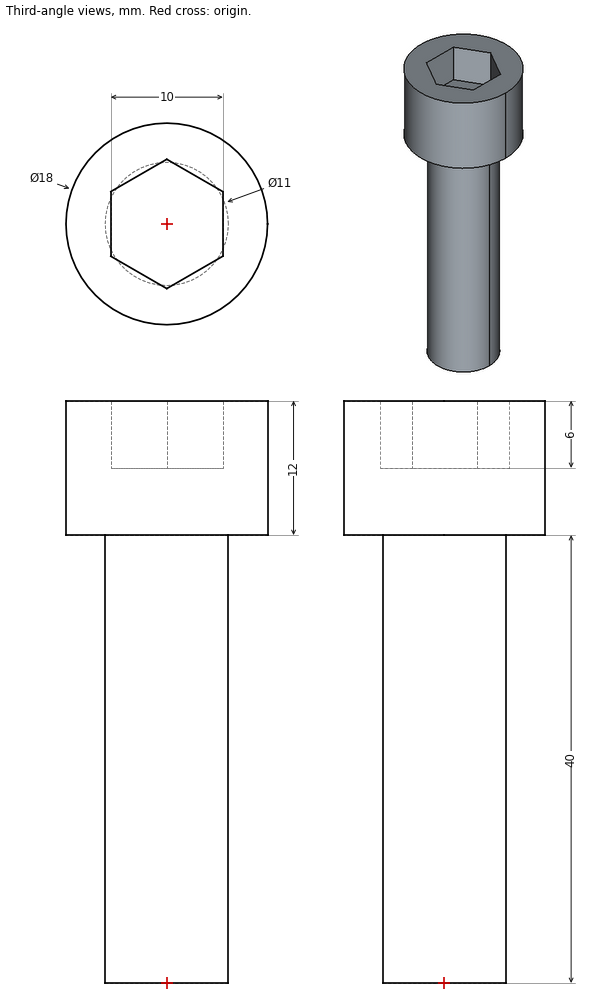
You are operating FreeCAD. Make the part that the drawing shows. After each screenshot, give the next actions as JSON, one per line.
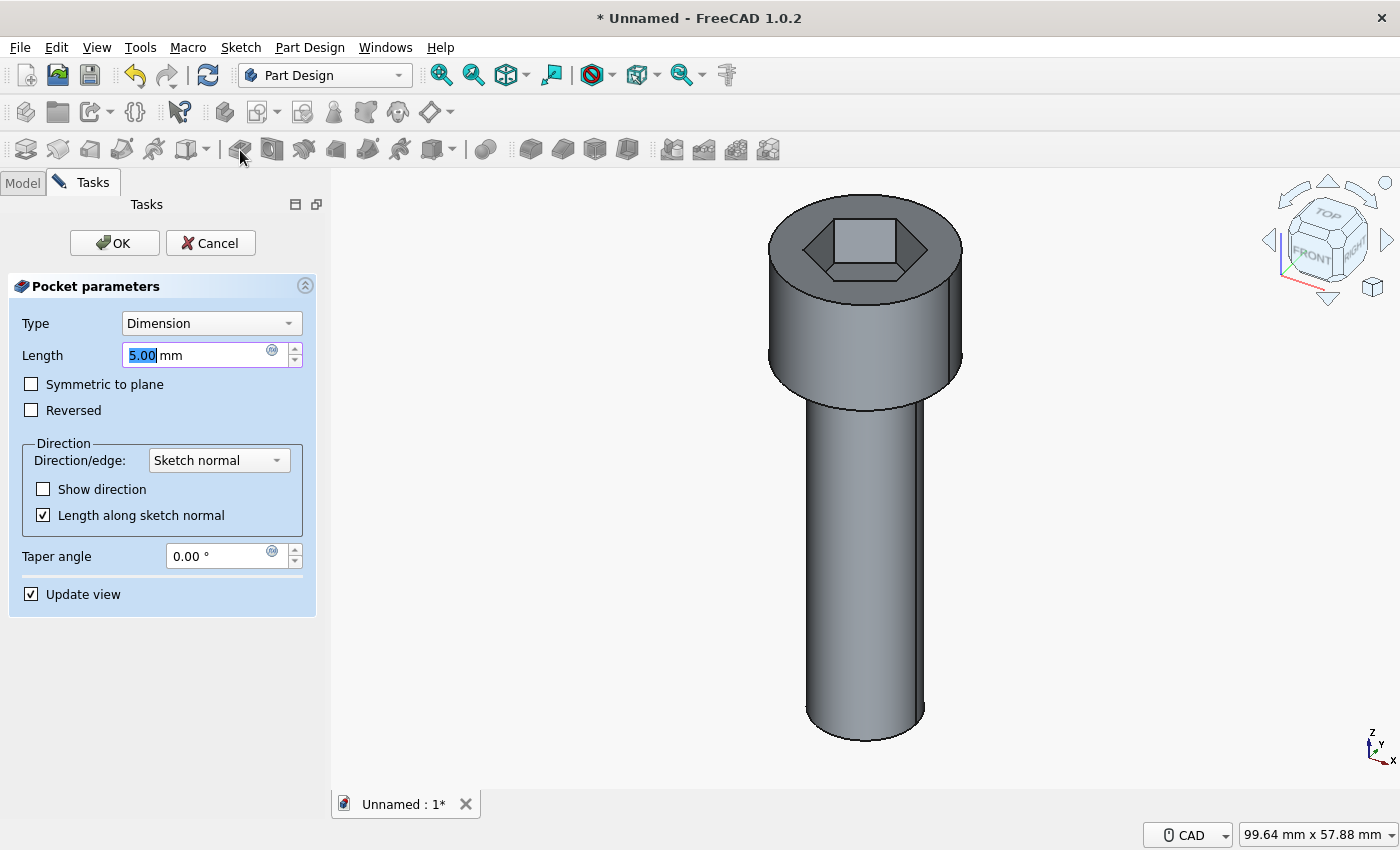
{"action": "type", "text": "6"}
{"action": "key", "text": "Tab"}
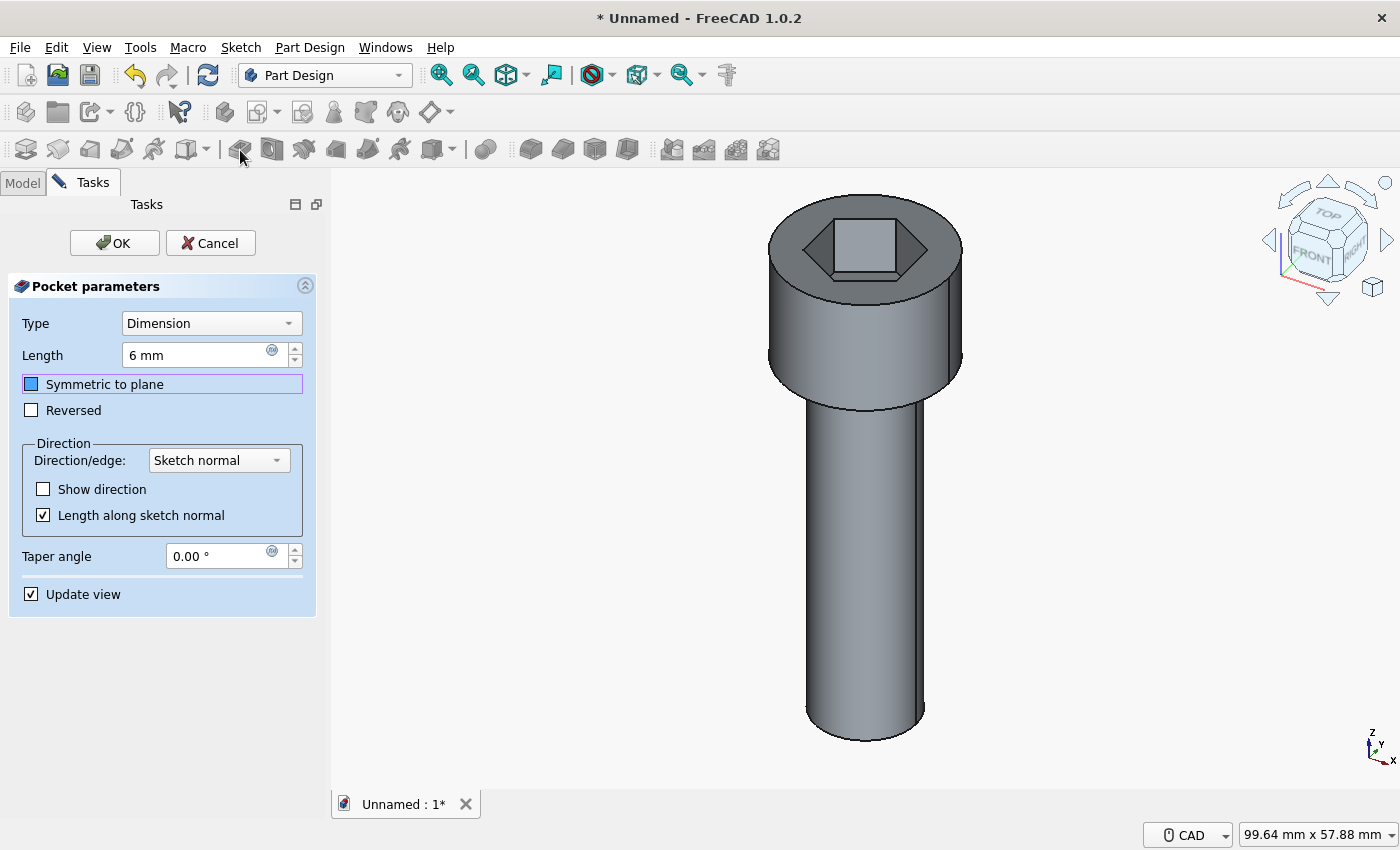
{"action": "left_click", "coordinate": [115, 243]}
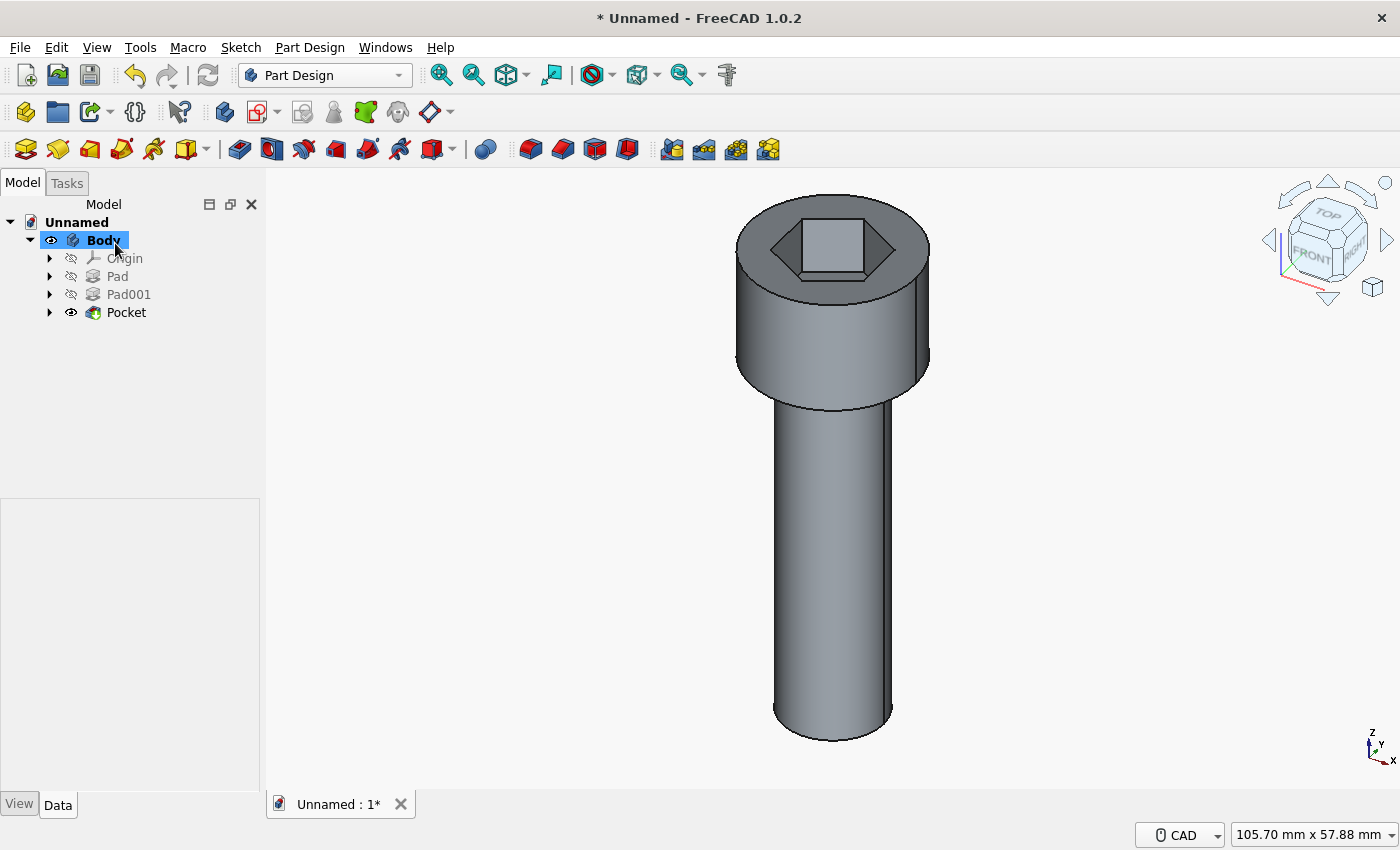
{"action": "key", "text": "0"}